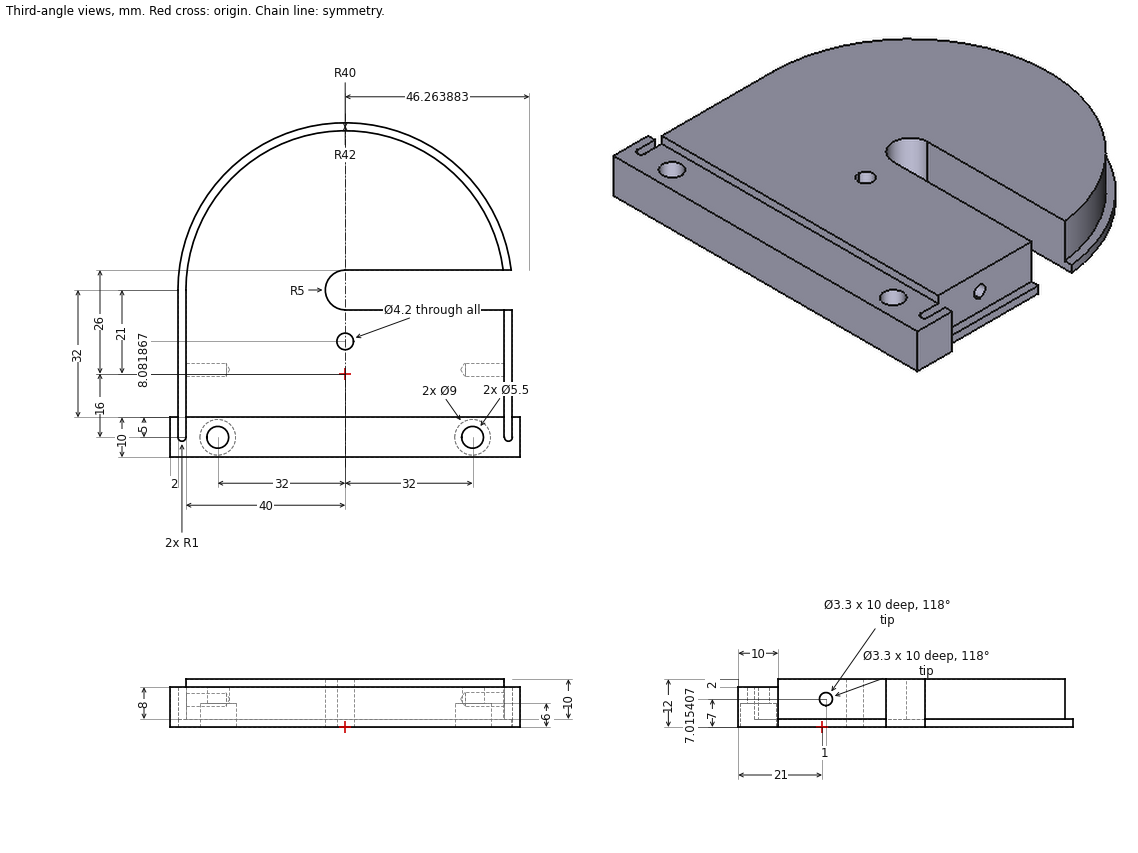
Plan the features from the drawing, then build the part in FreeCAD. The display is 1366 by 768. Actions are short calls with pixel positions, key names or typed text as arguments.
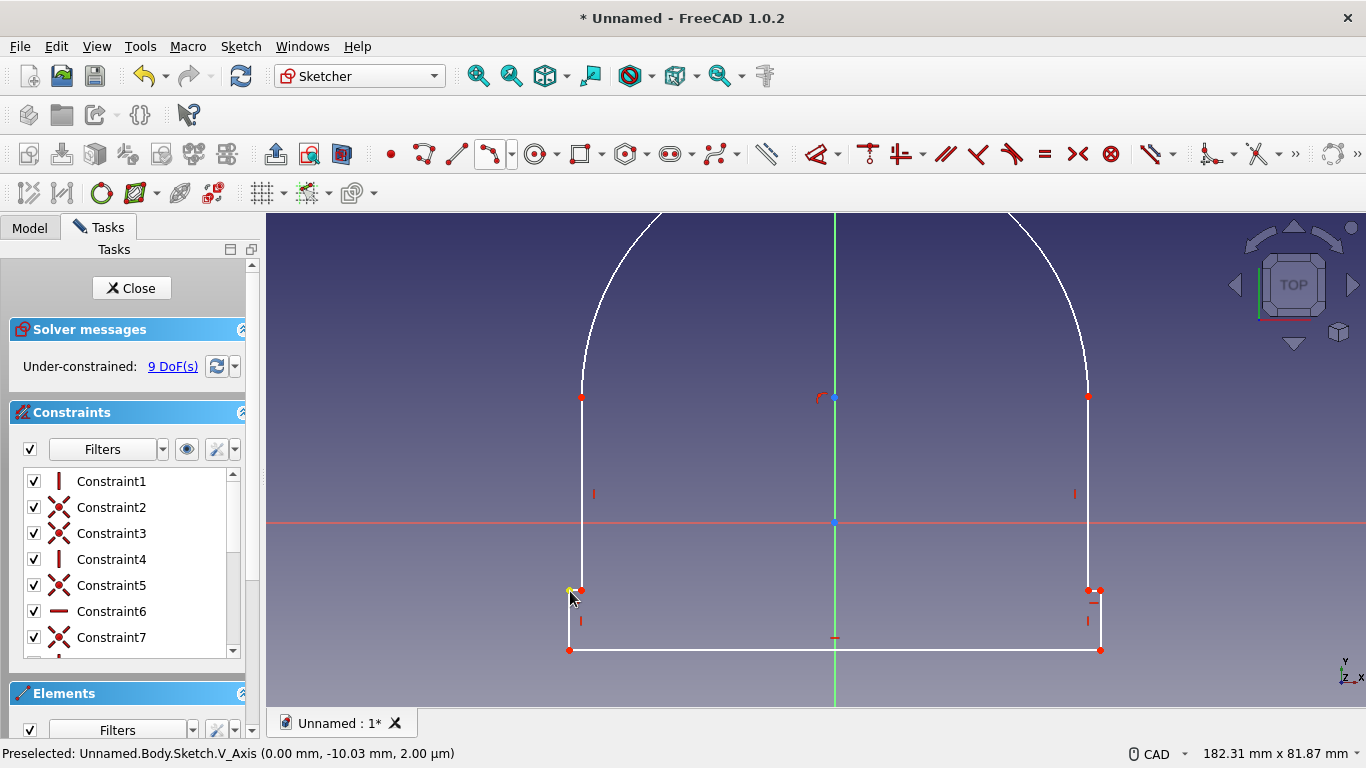
click(569, 590)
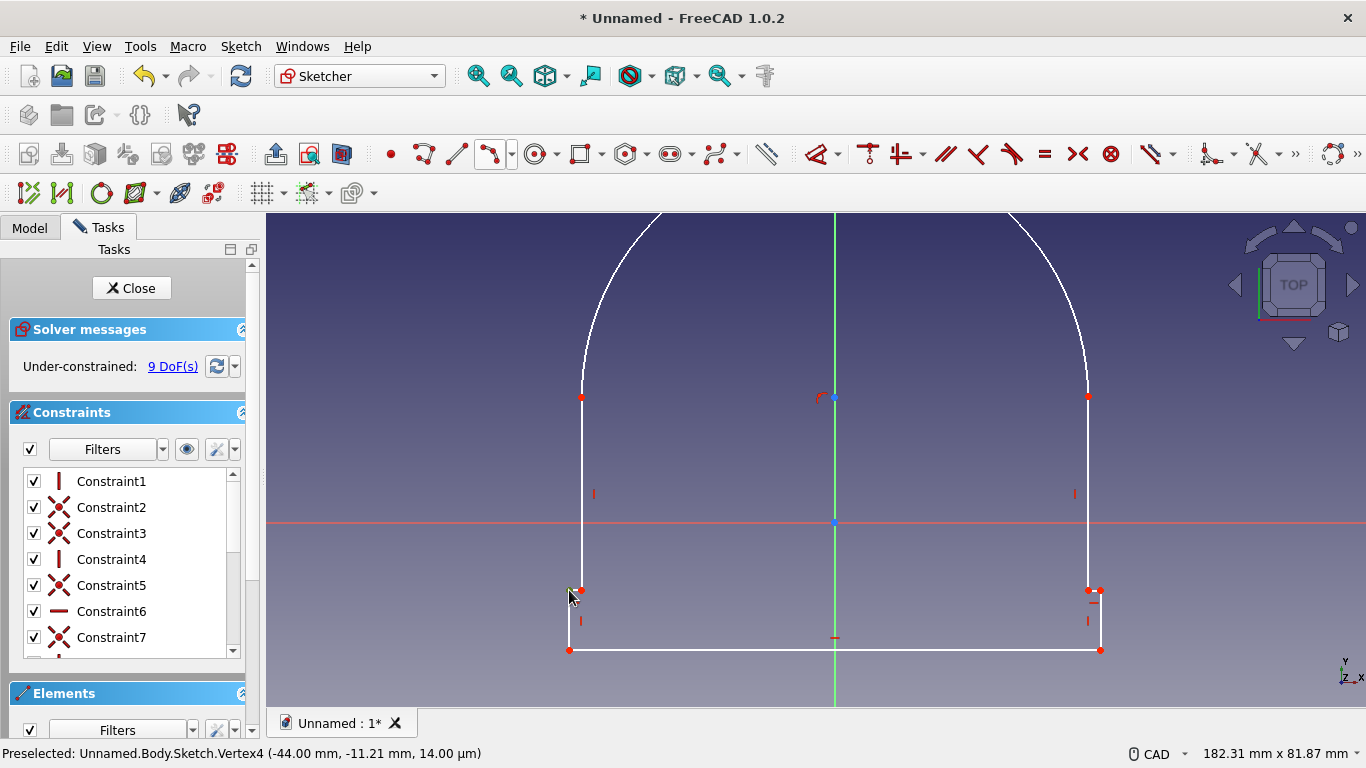
click(1101, 591)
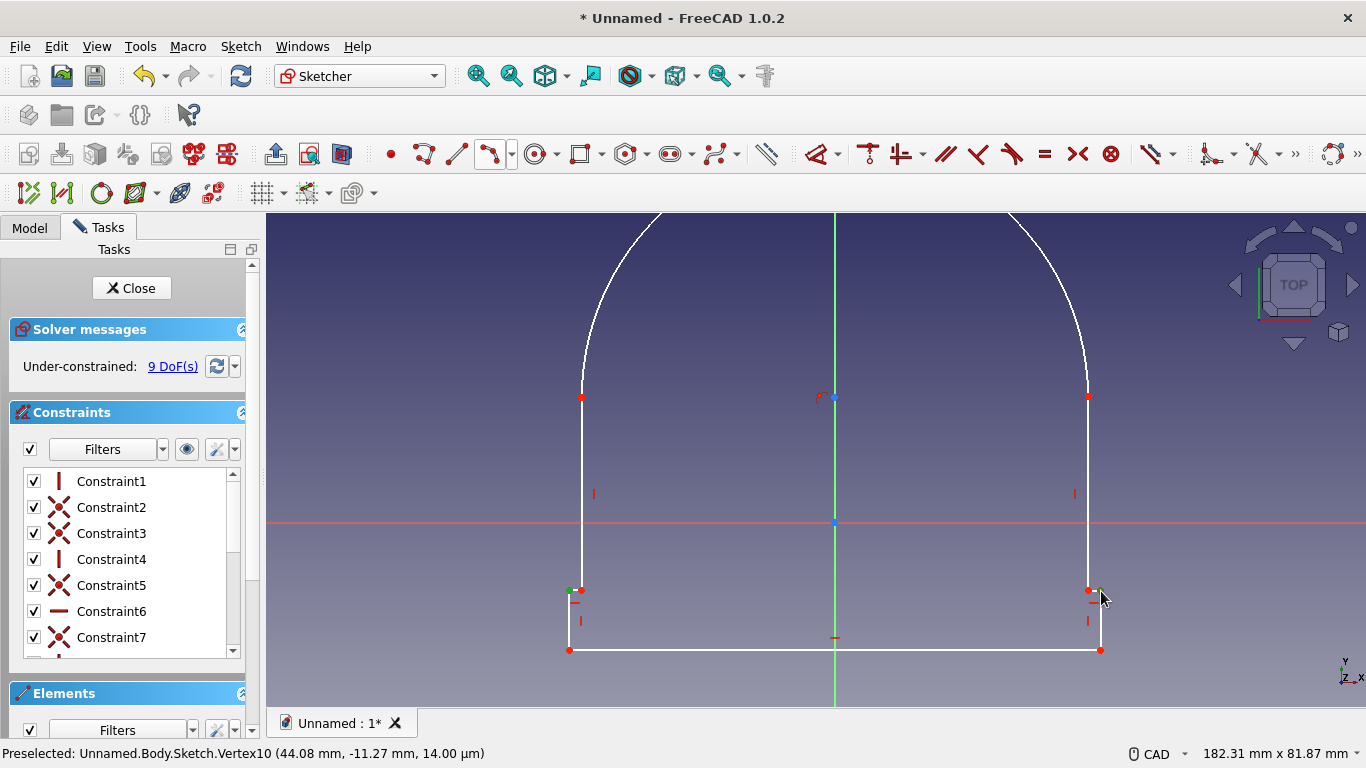
click(835, 616)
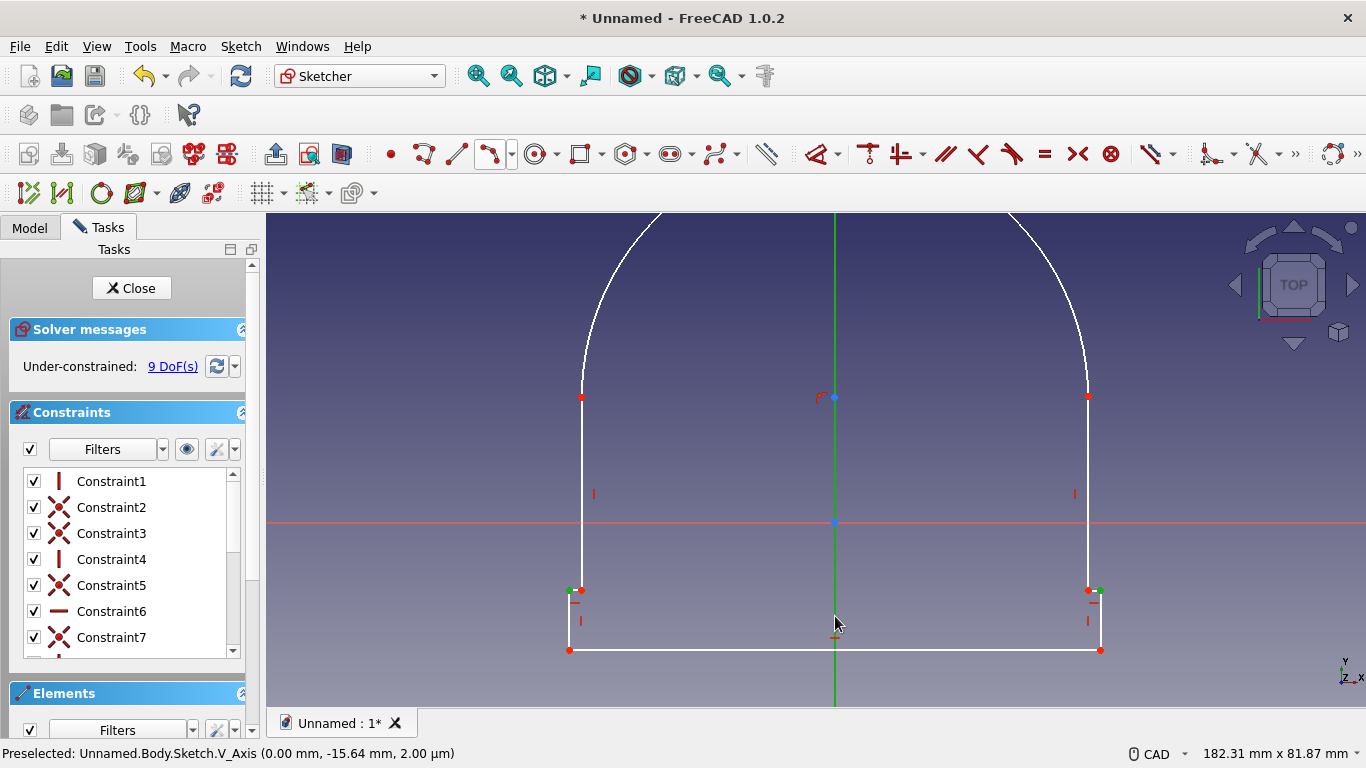
click(1078, 154)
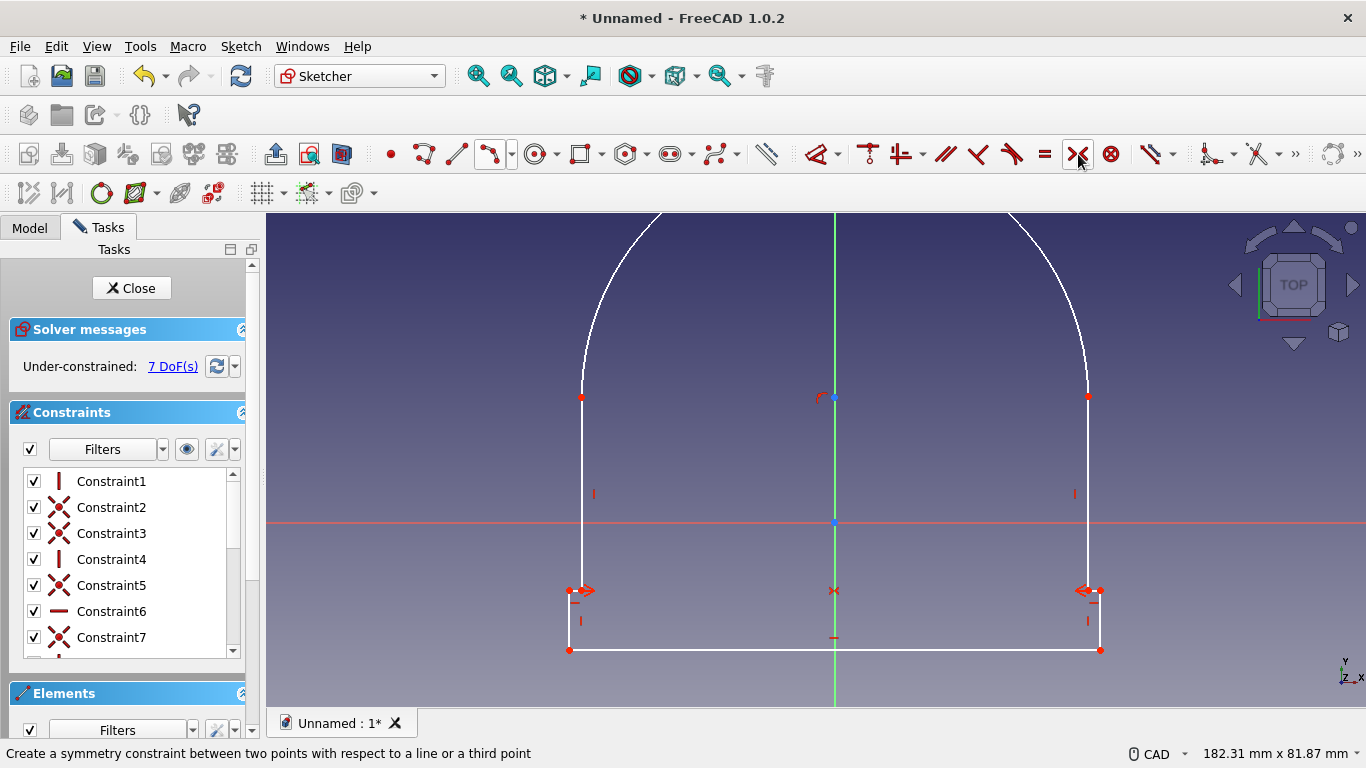
click(816, 154)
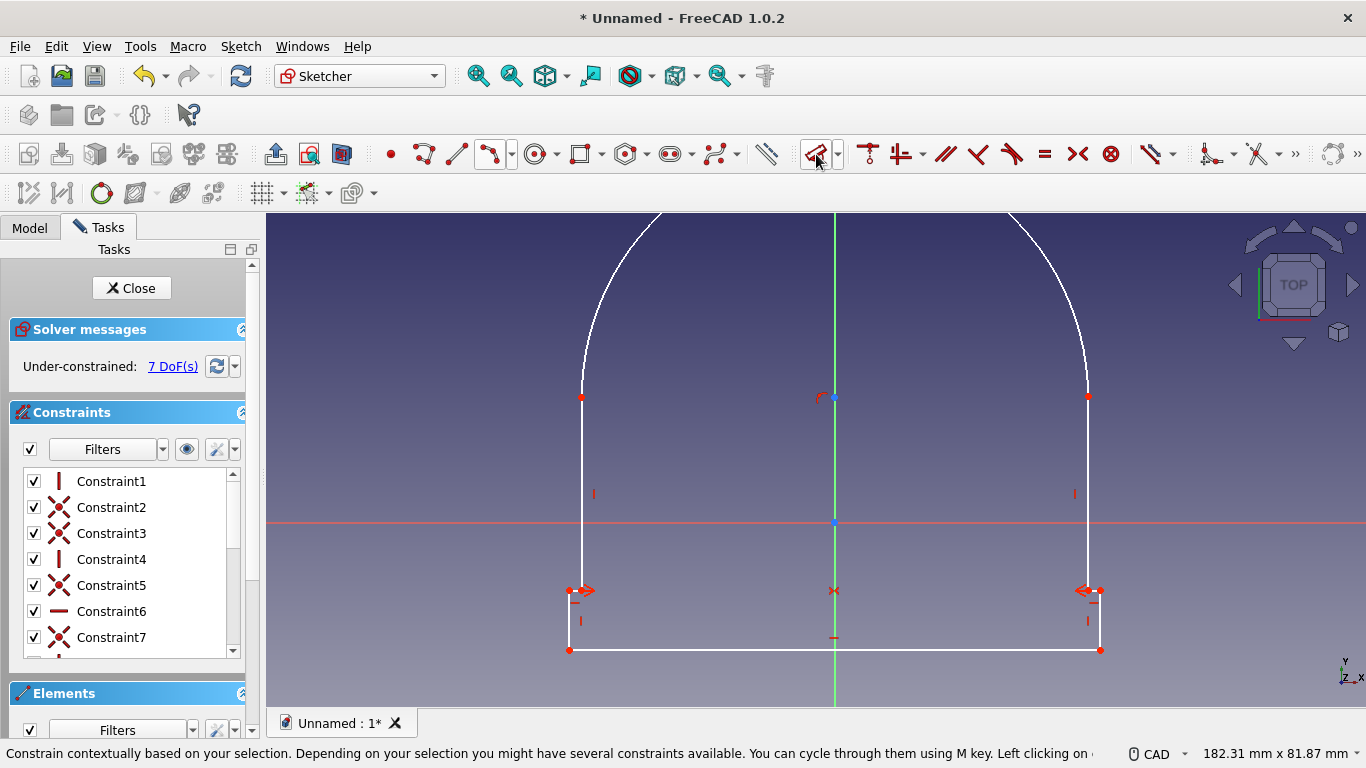
click(1039, 248)
click(1118, 360)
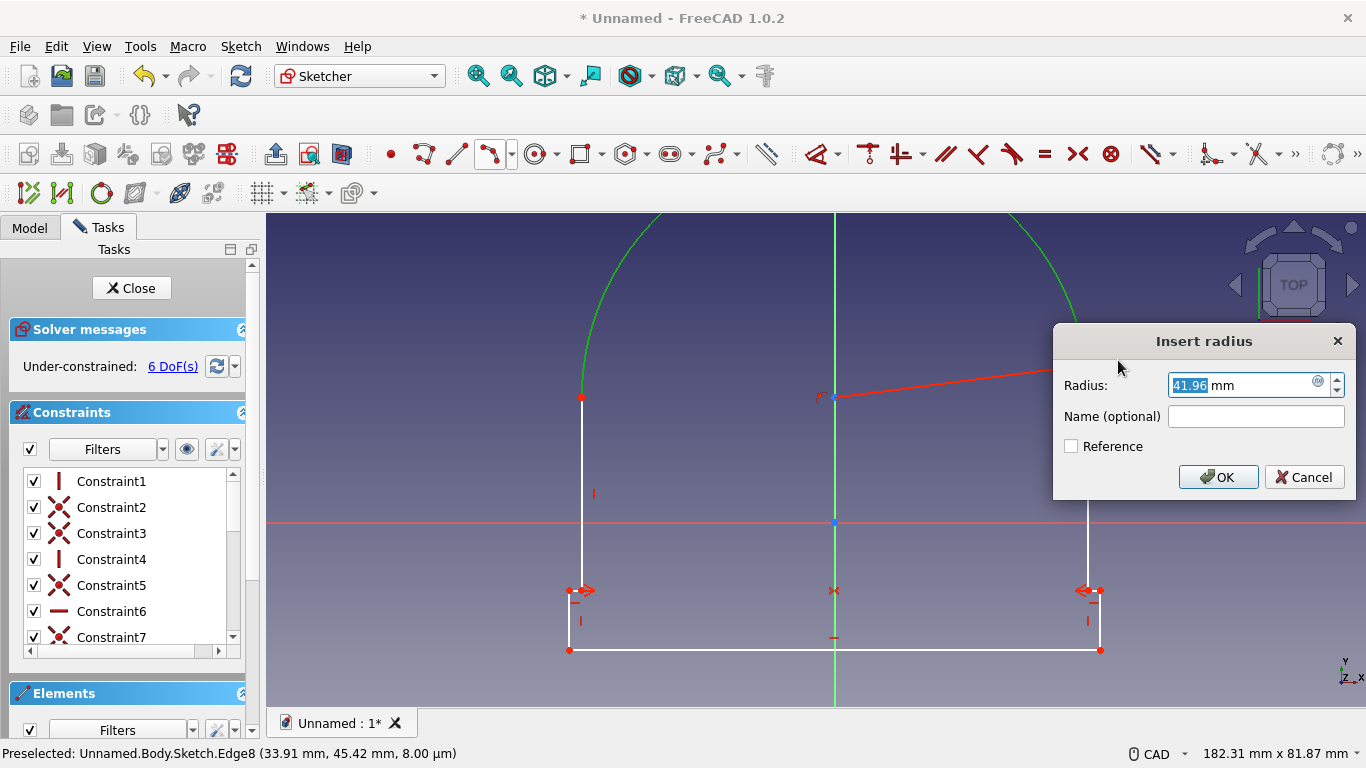
text(42)
key(Return)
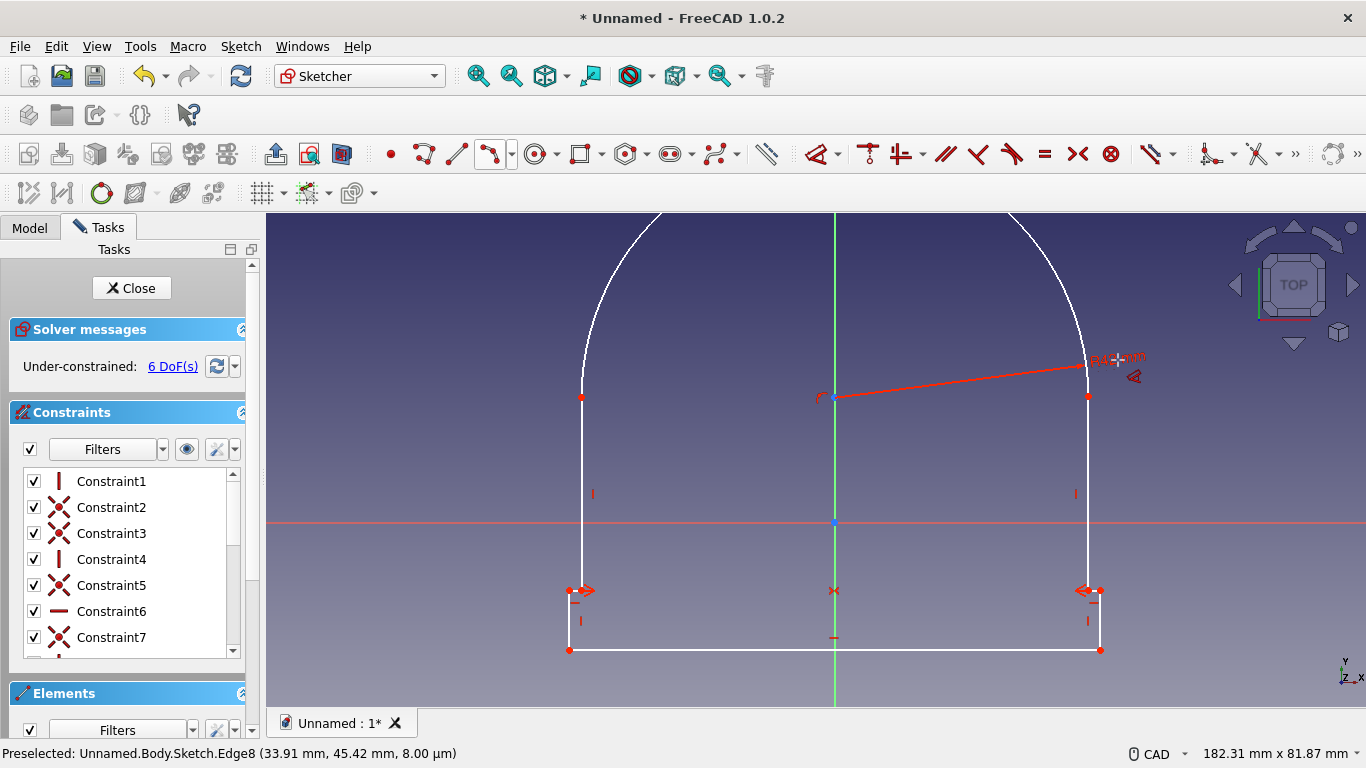
scroll(576, 591, up, 6)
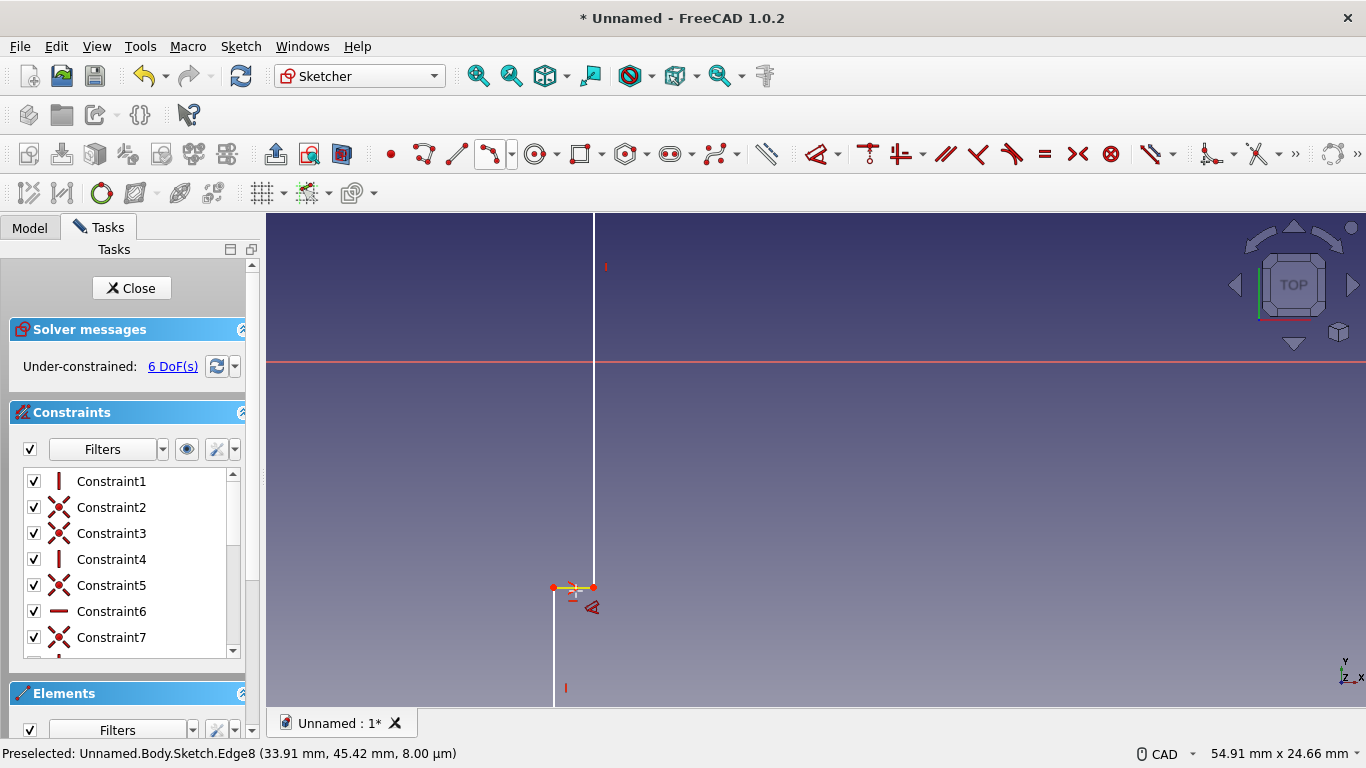
click(574, 588)
click(574, 622)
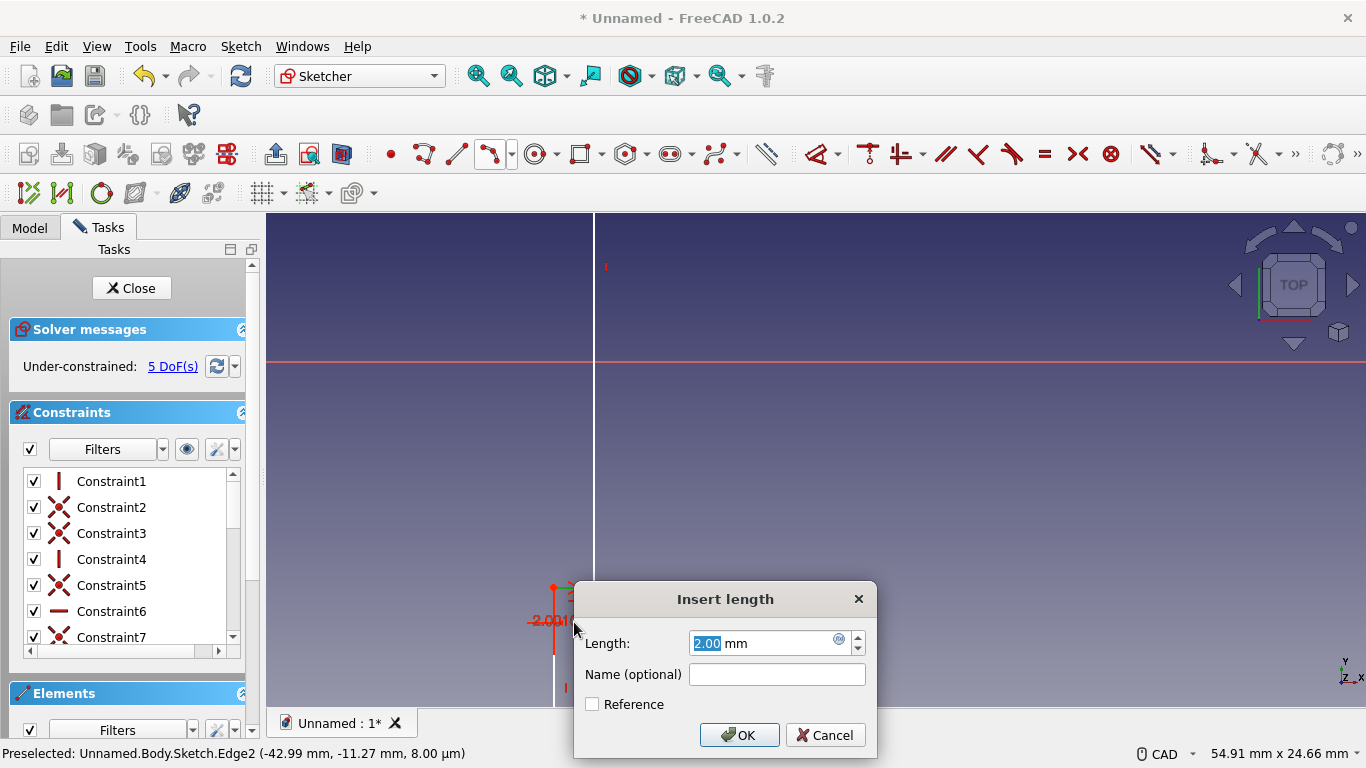
text(2)
key(Return)